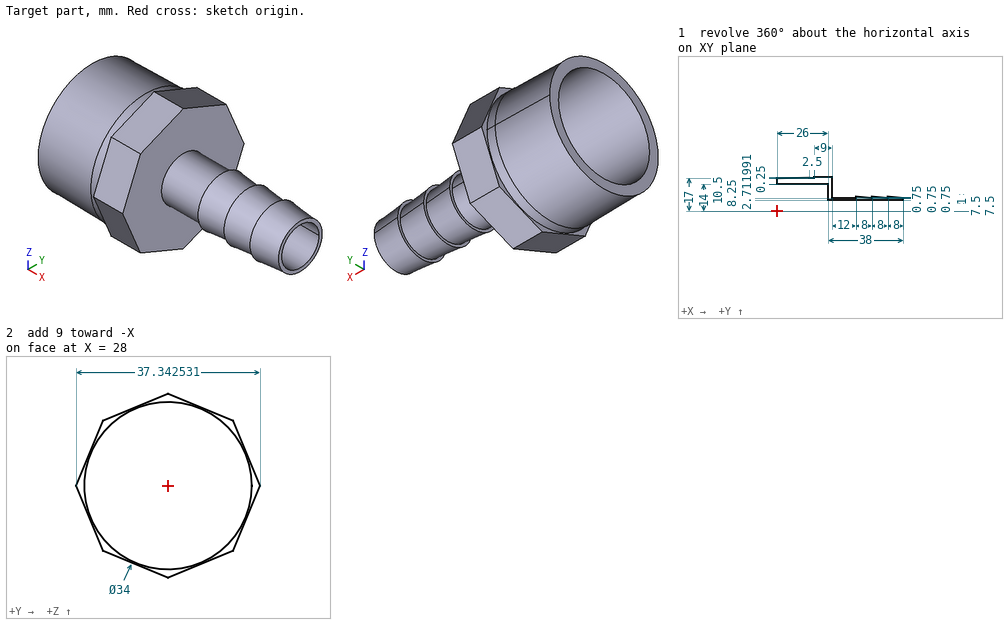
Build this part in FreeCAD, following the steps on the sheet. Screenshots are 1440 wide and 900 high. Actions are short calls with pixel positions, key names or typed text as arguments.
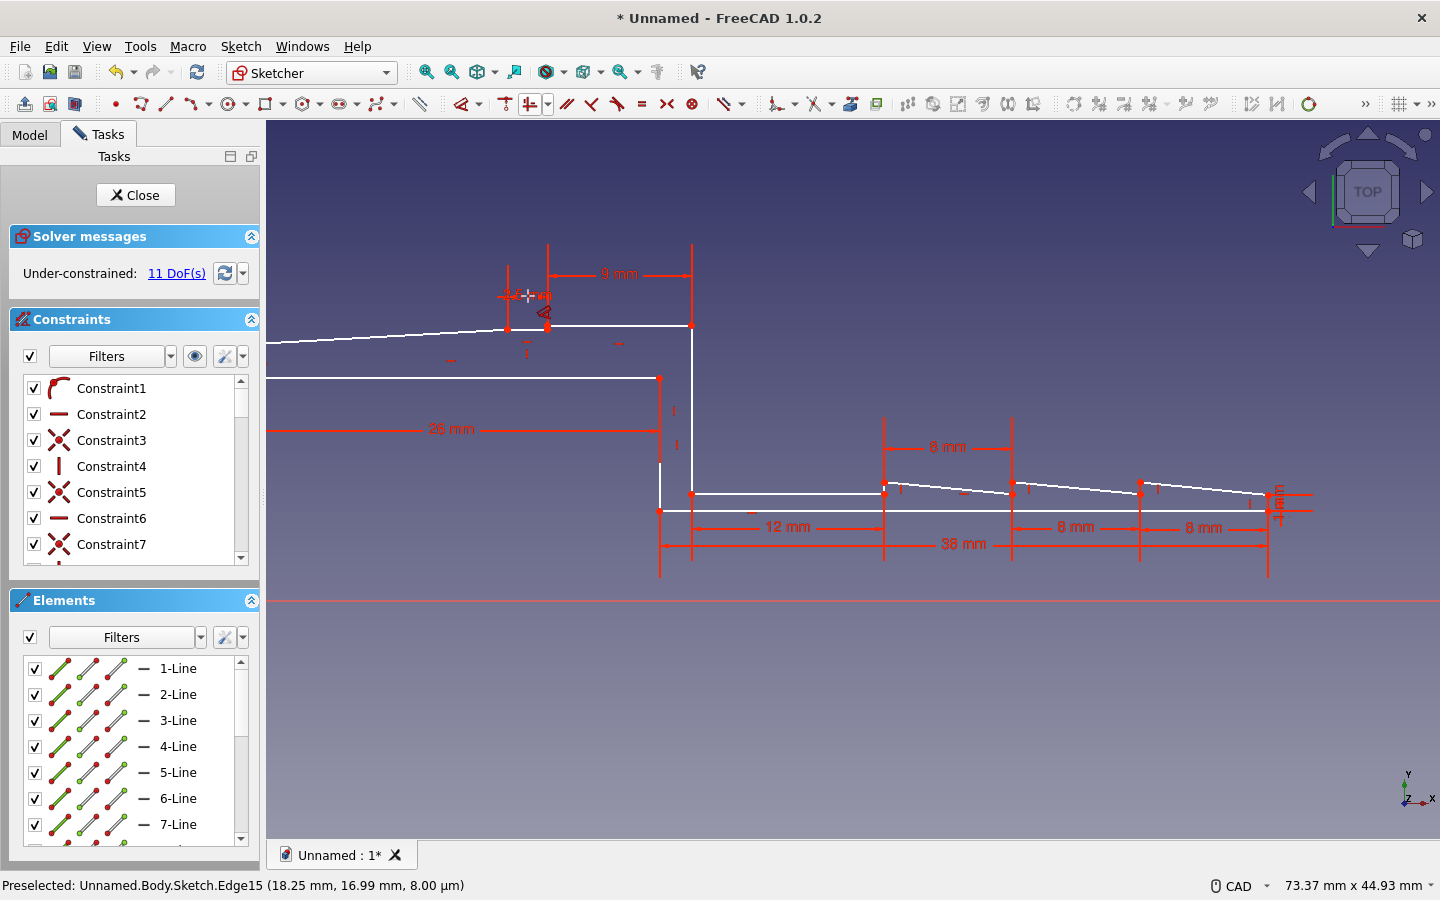
scroll(842, 512, down, 2)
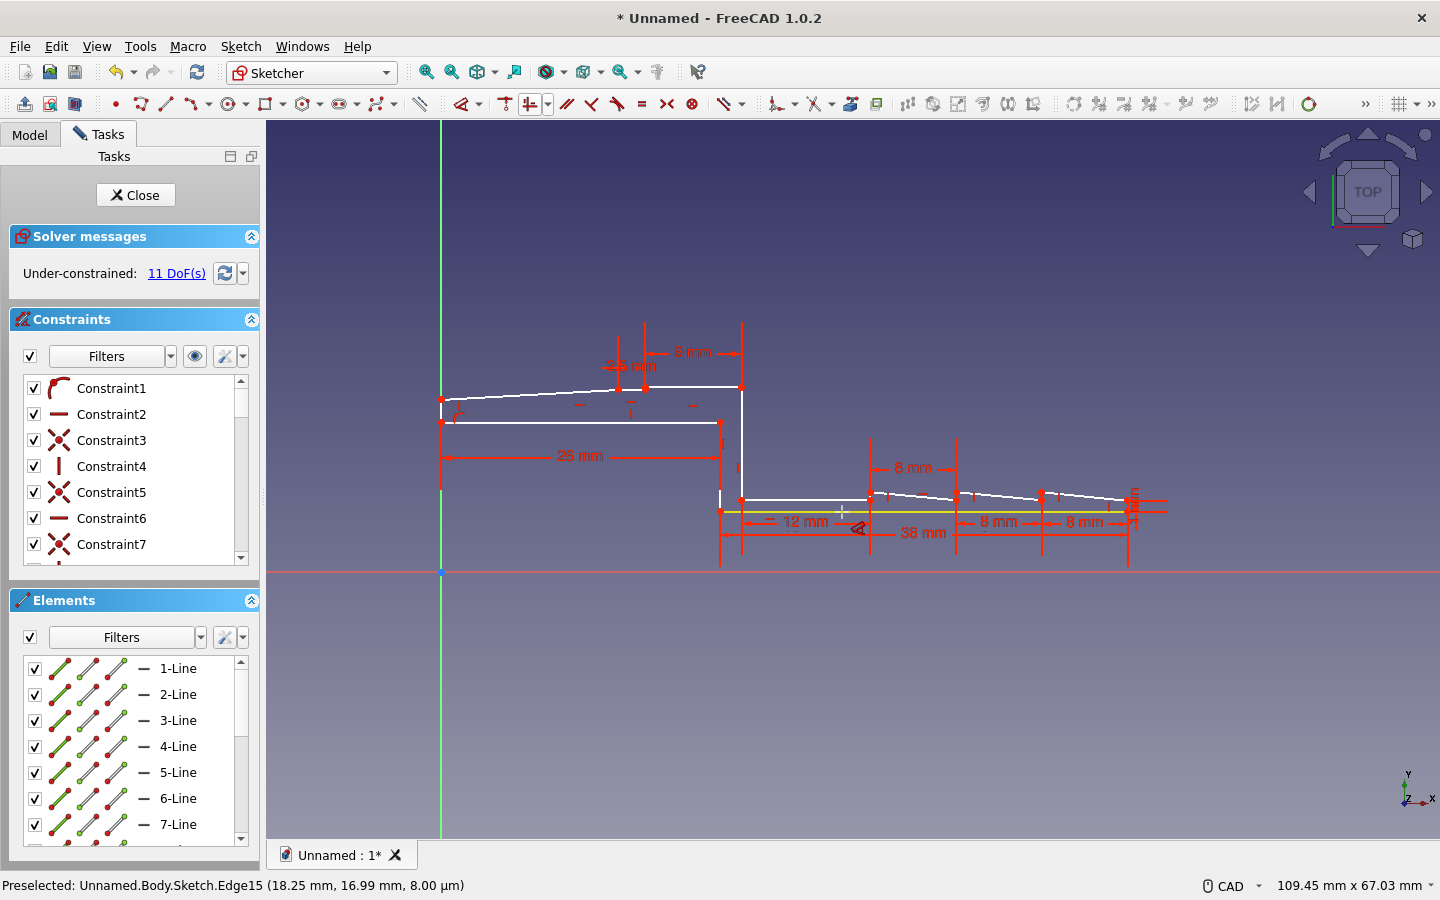
click(441, 423)
click(407, 497)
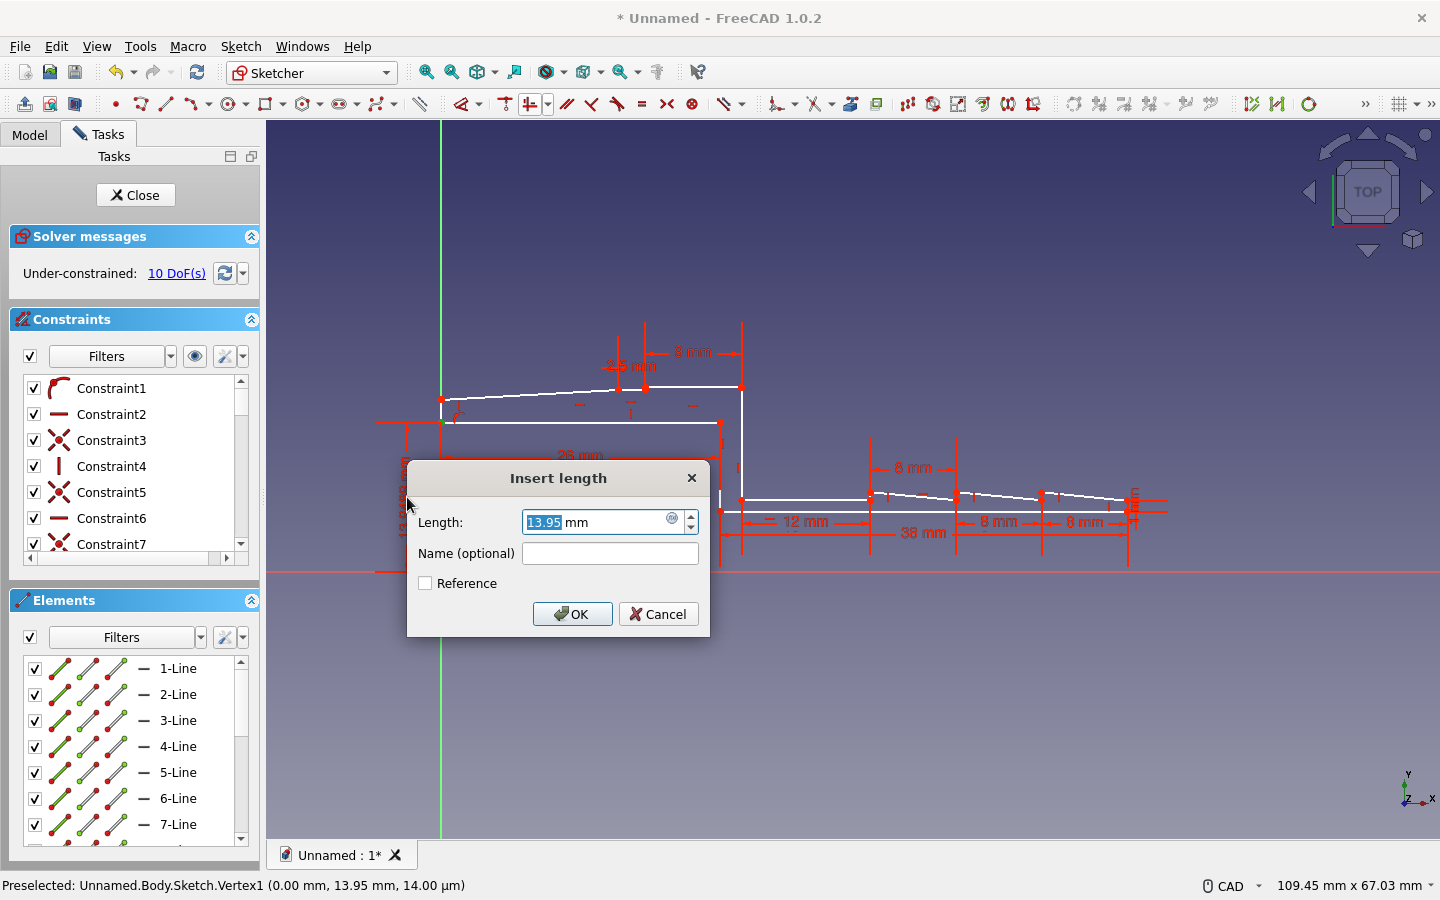
text(14)
key(Return)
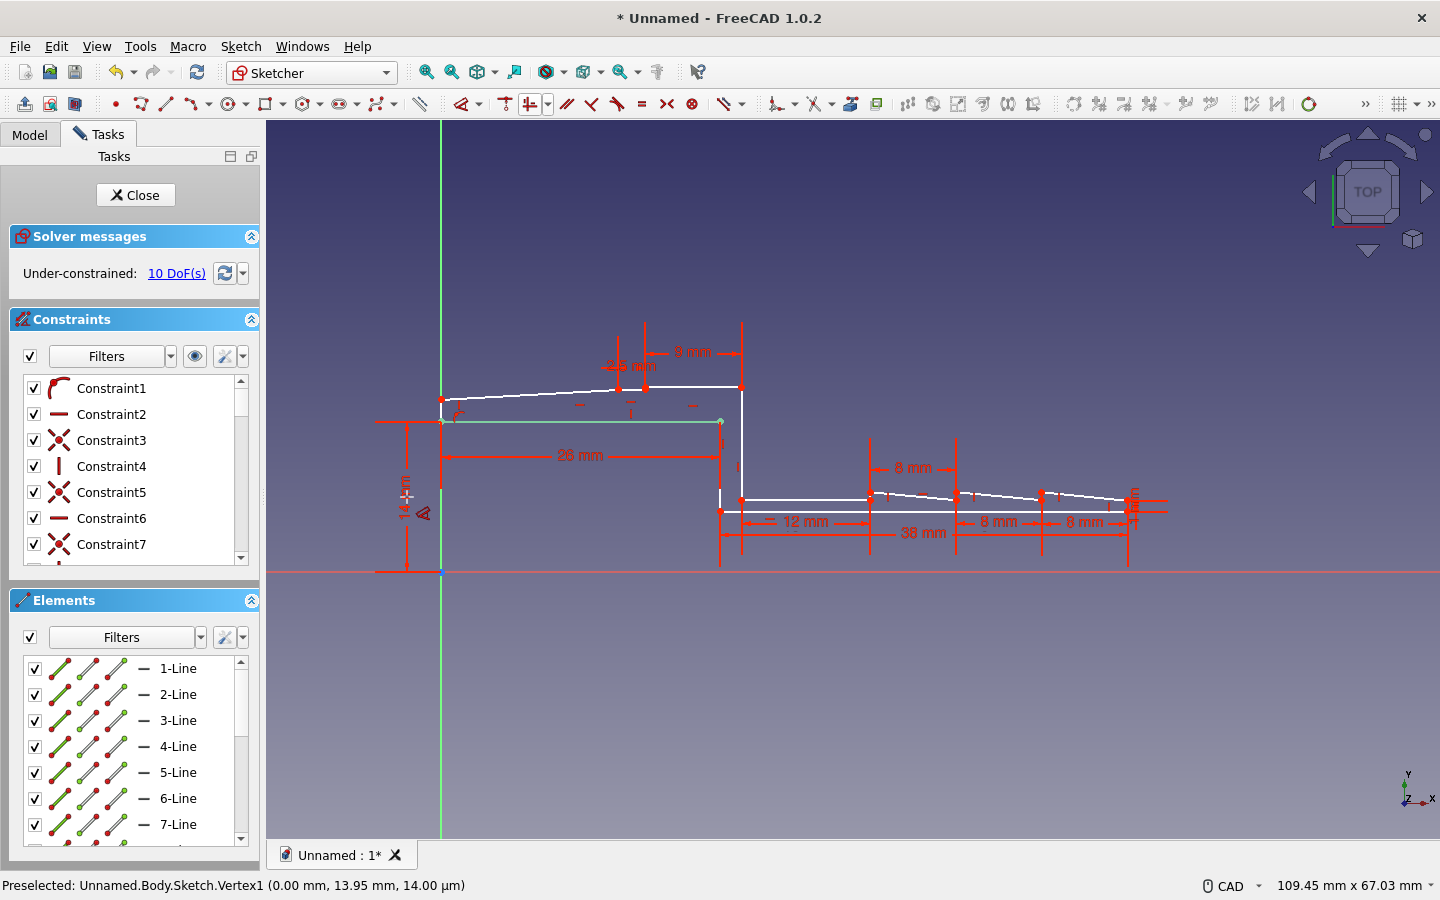
scroll(645, 390, up, 8)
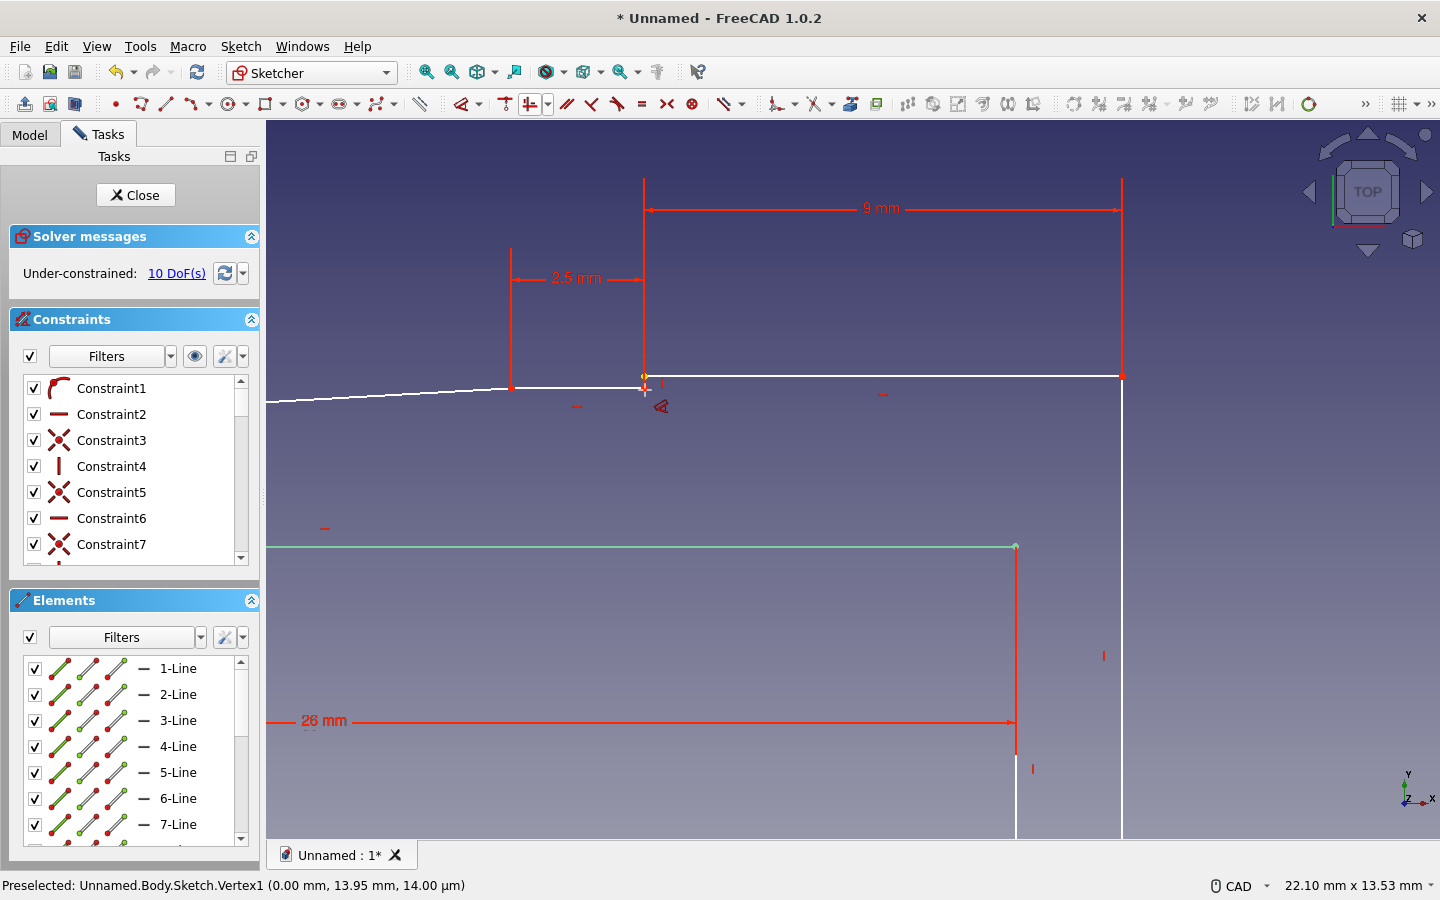
click(644, 388)
click(678, 600)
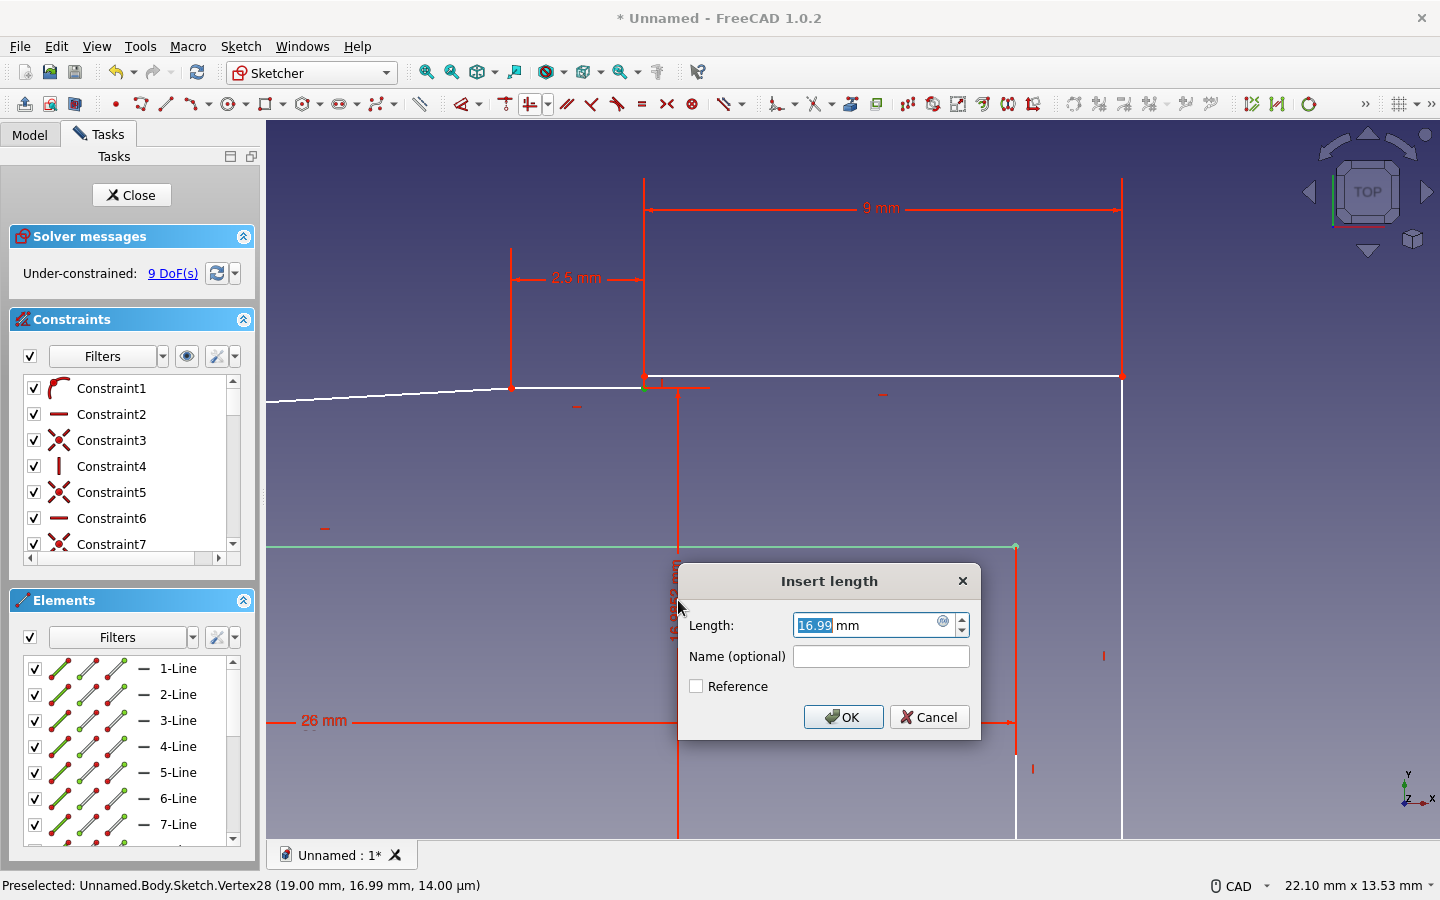
text(17)
key(Return)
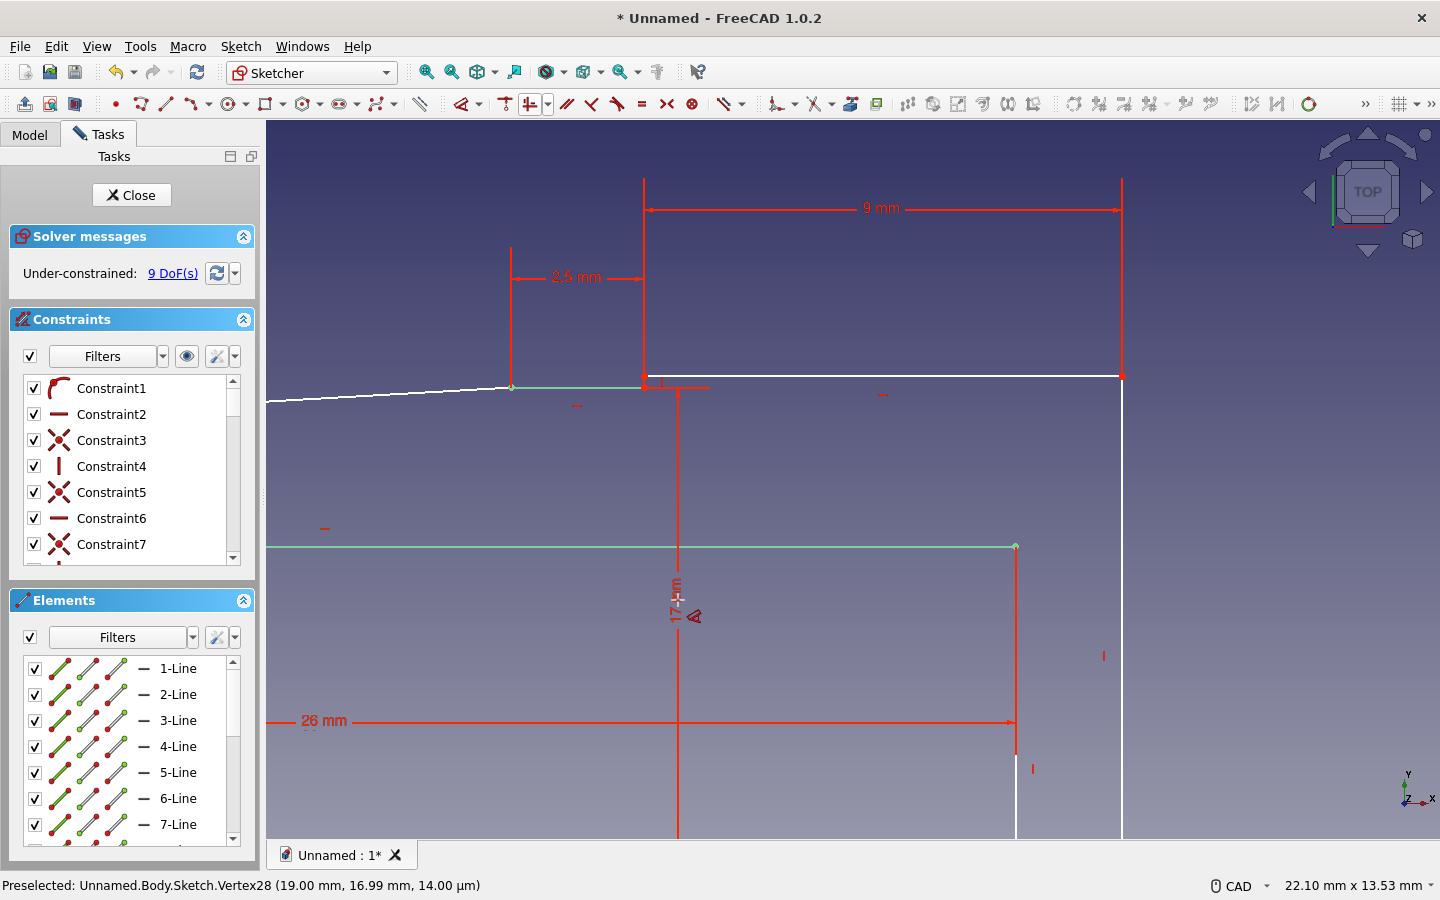
scroll(645, 390, down, 8)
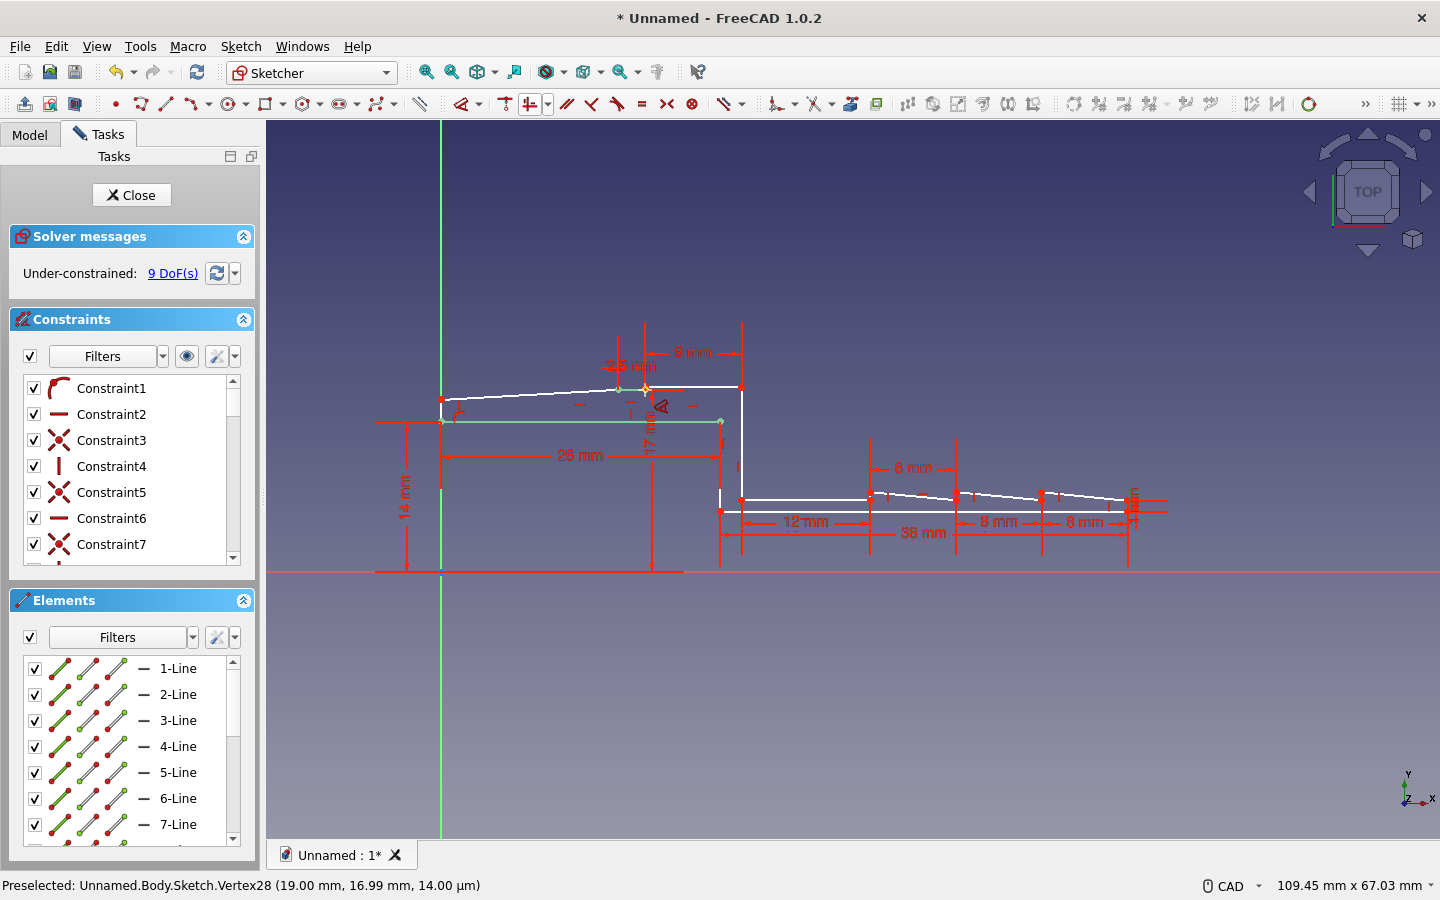
click(720, 449)
click(686, 467)